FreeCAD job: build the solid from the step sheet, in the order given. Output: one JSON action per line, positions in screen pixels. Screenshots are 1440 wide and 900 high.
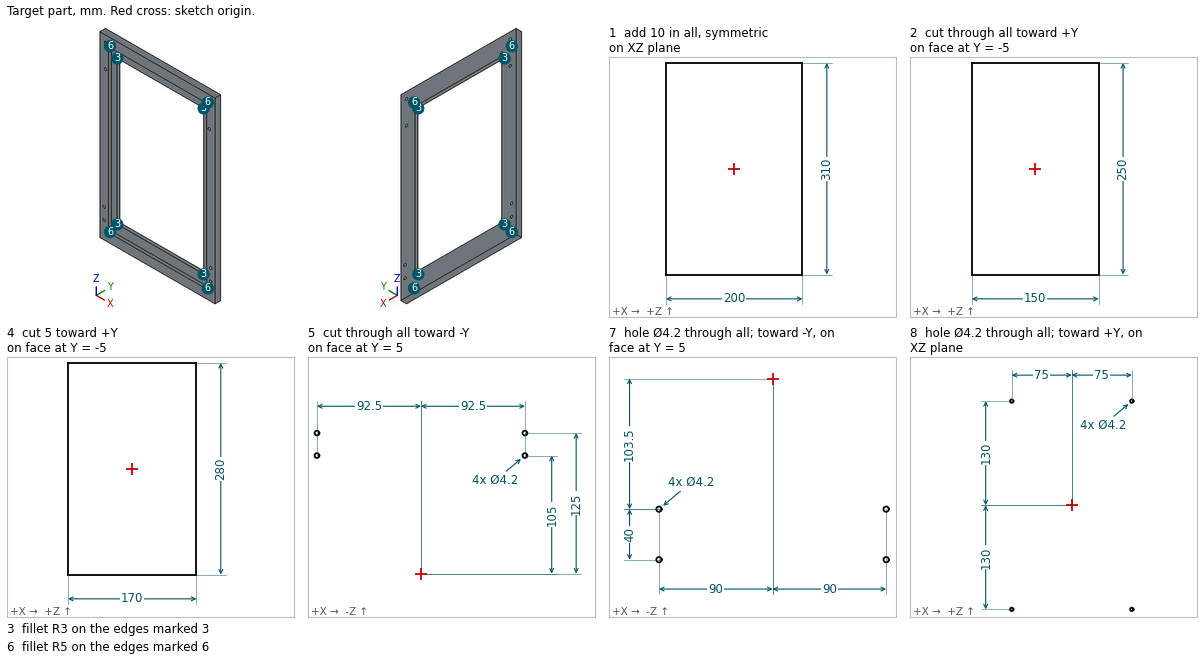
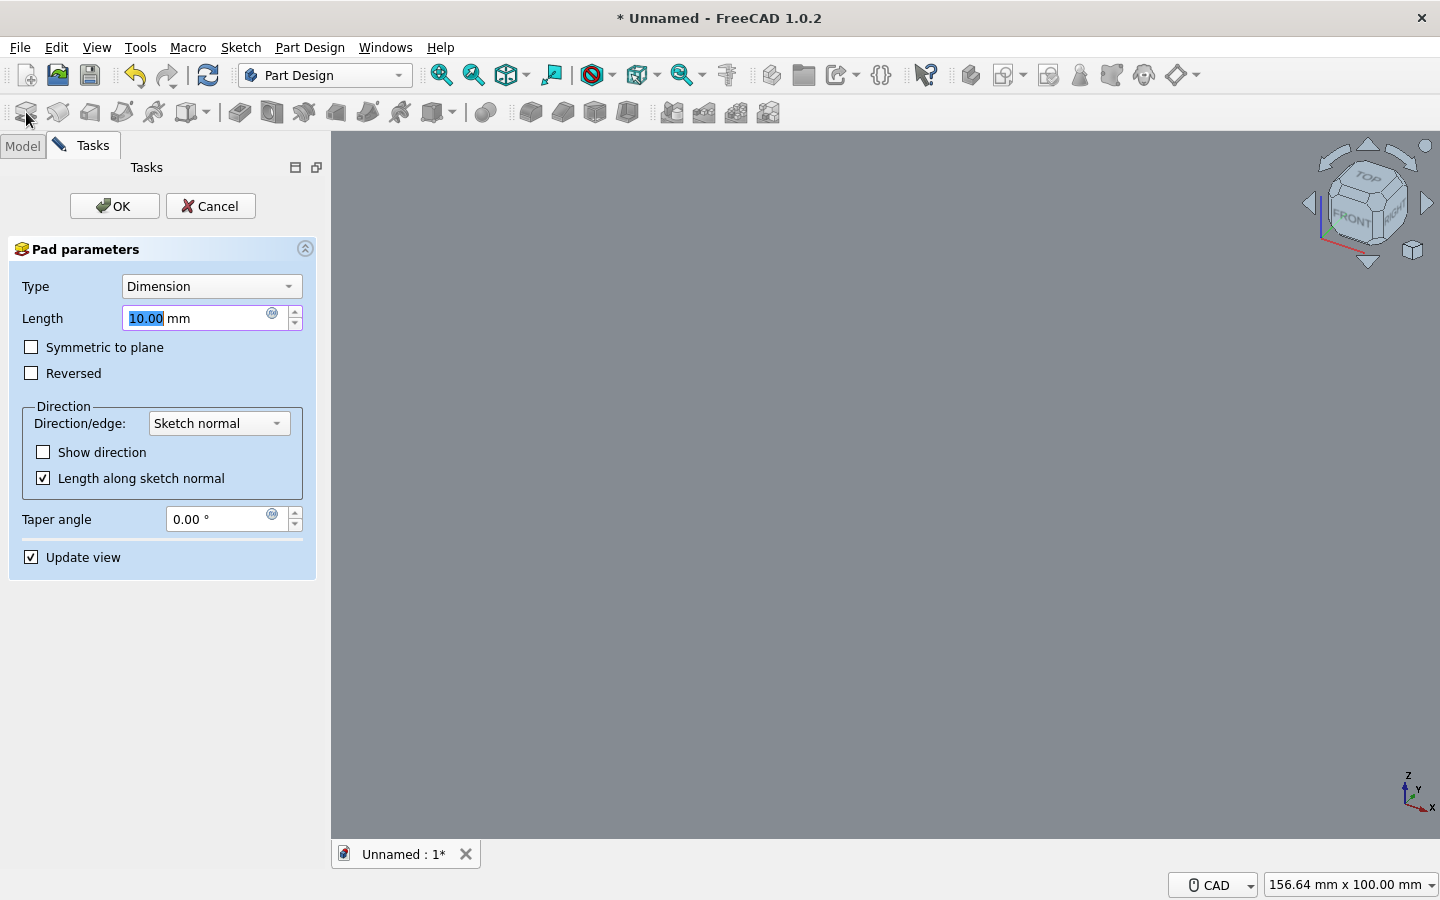
{"action": "type", "text": "10"}
{"action": "key", "text": "Tab"}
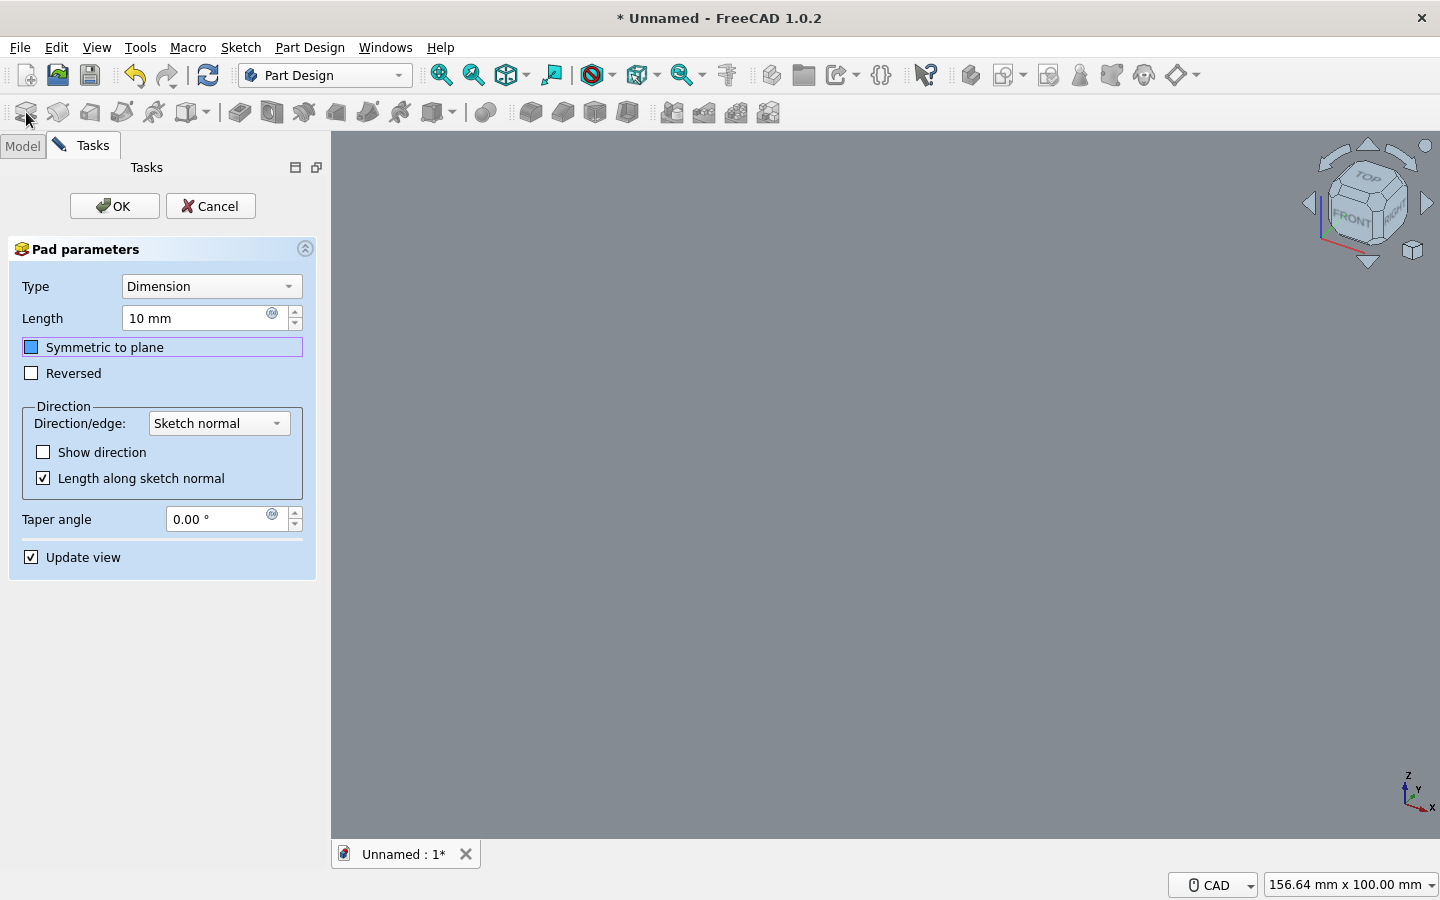
{"action": "left_click", "coordinate": [30, 347]}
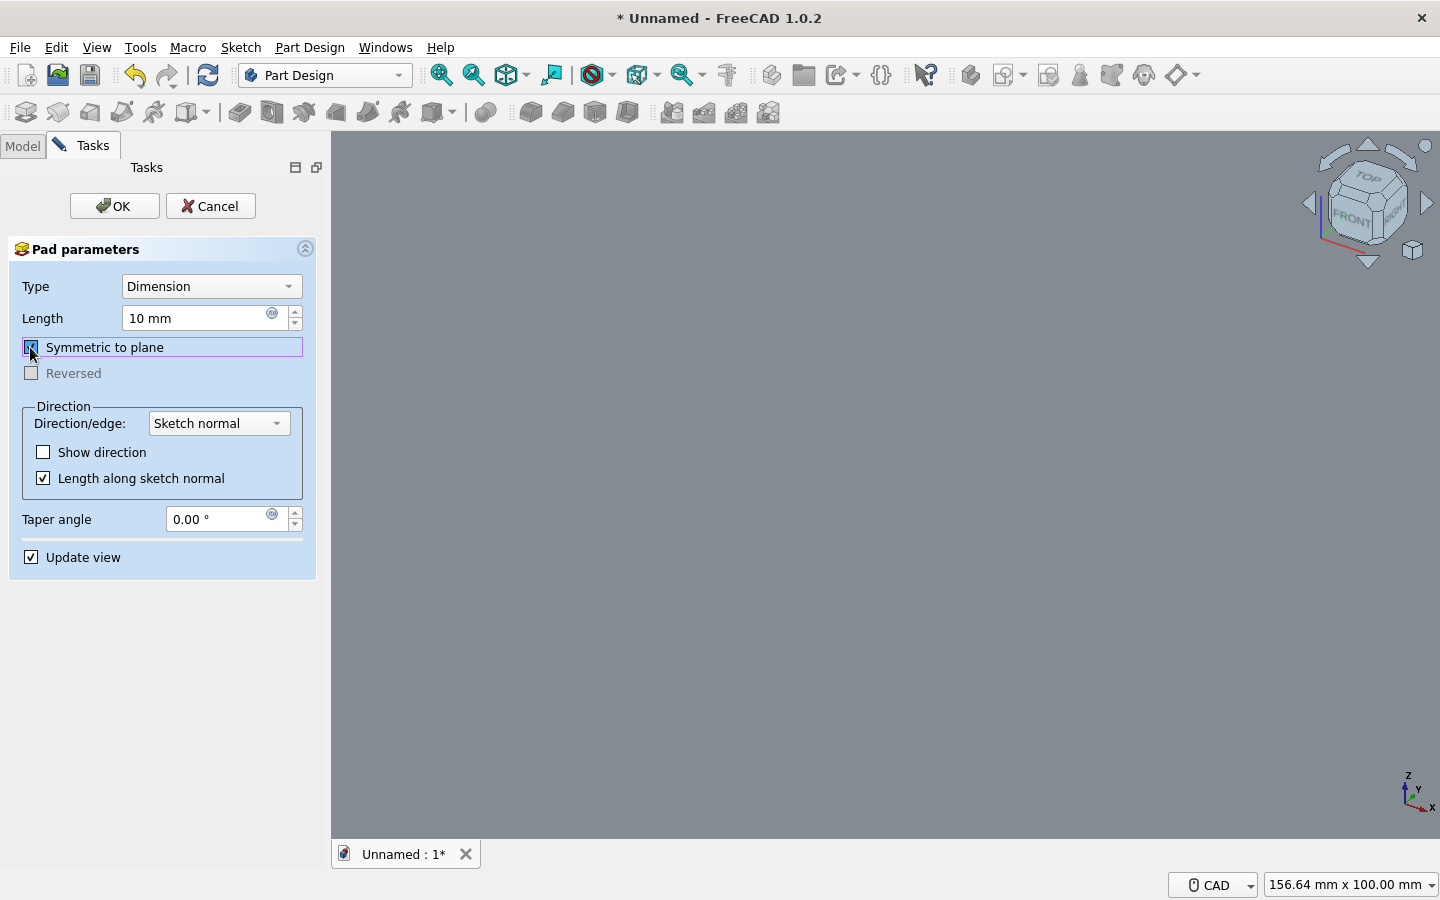
{"action": "left_click", "coordinate": [115, 206]}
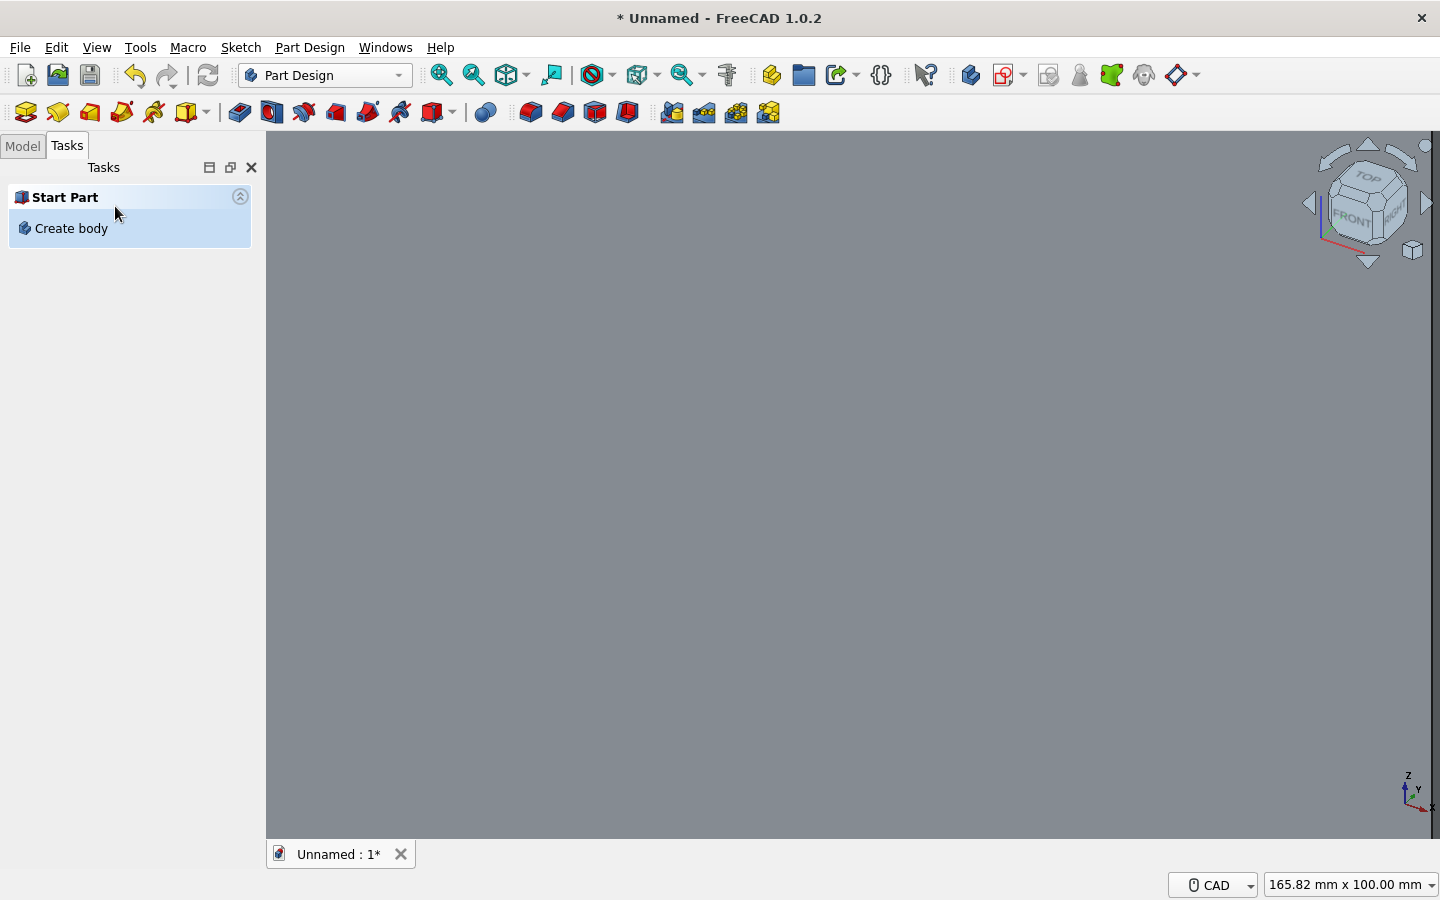
{"action": "left_click", "coordinate": [442, 76]}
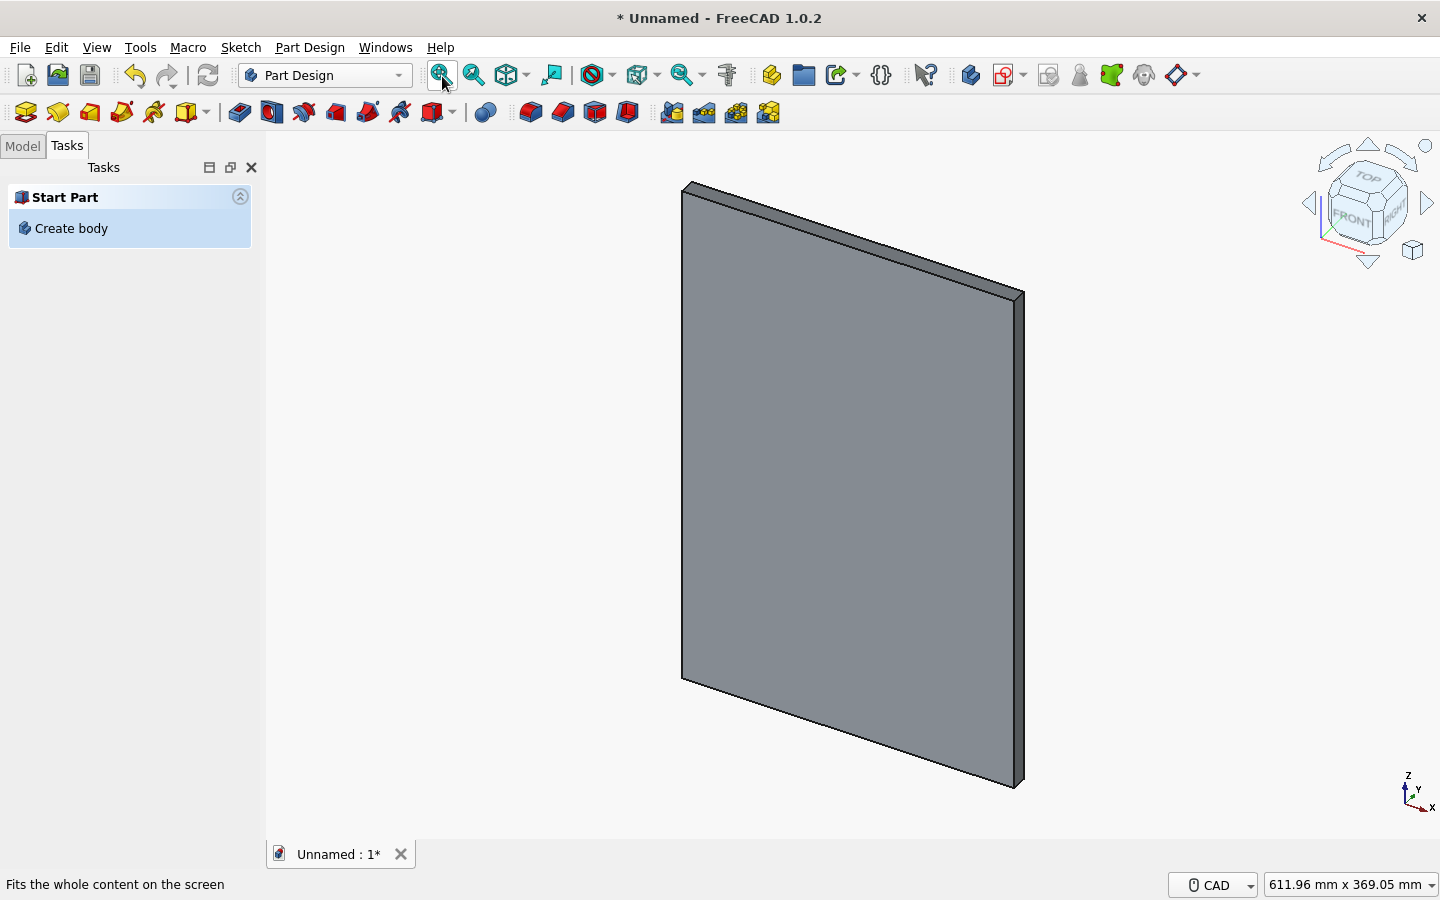
{"action": "left_click", "coordinate": [848, 419]}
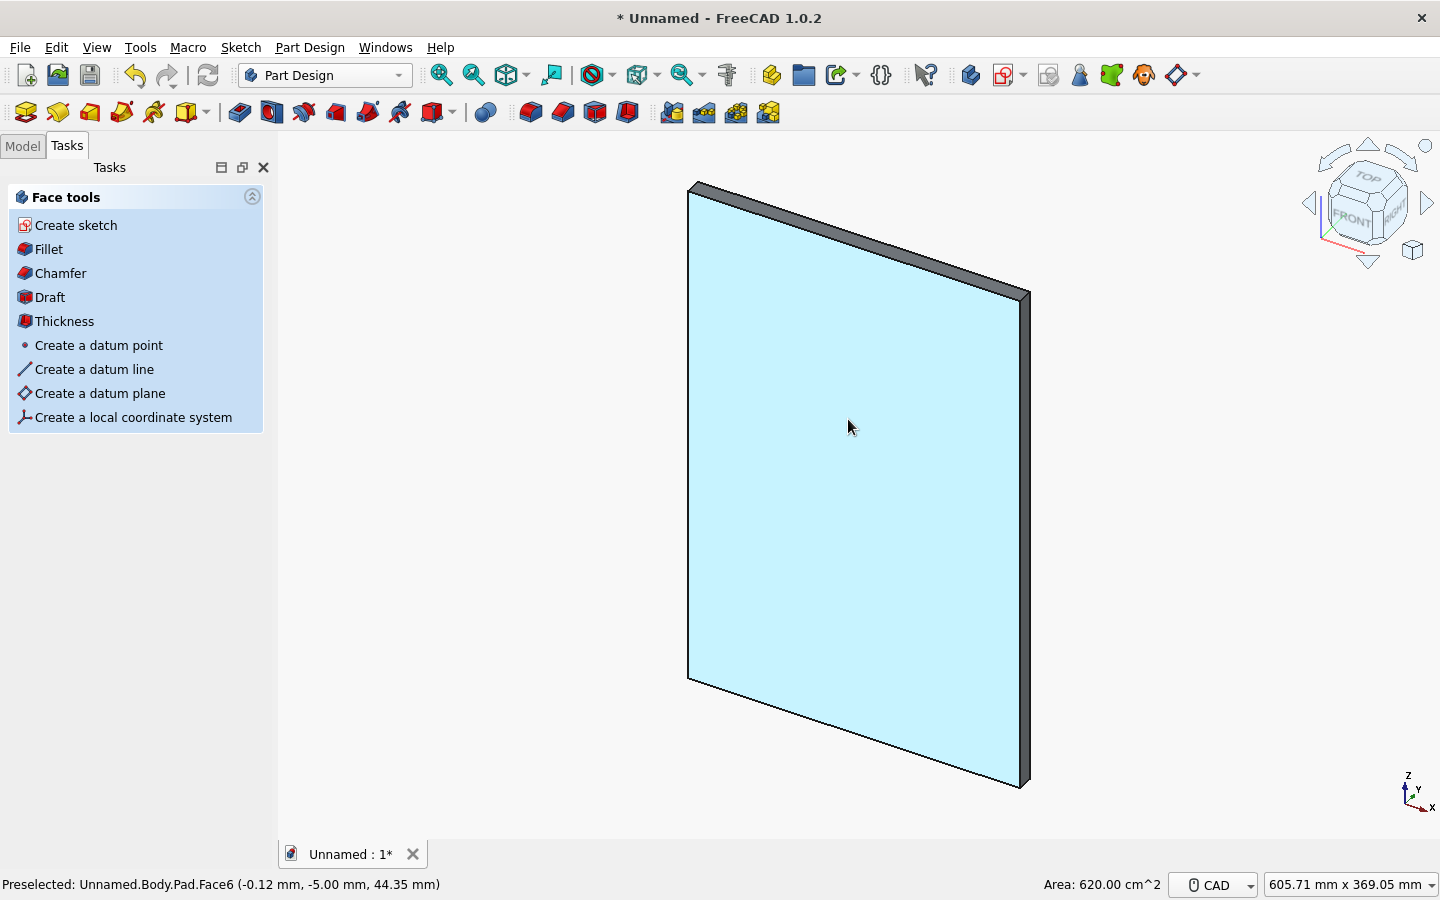
{"action": "left_click", "coordinate": [1004, 76]}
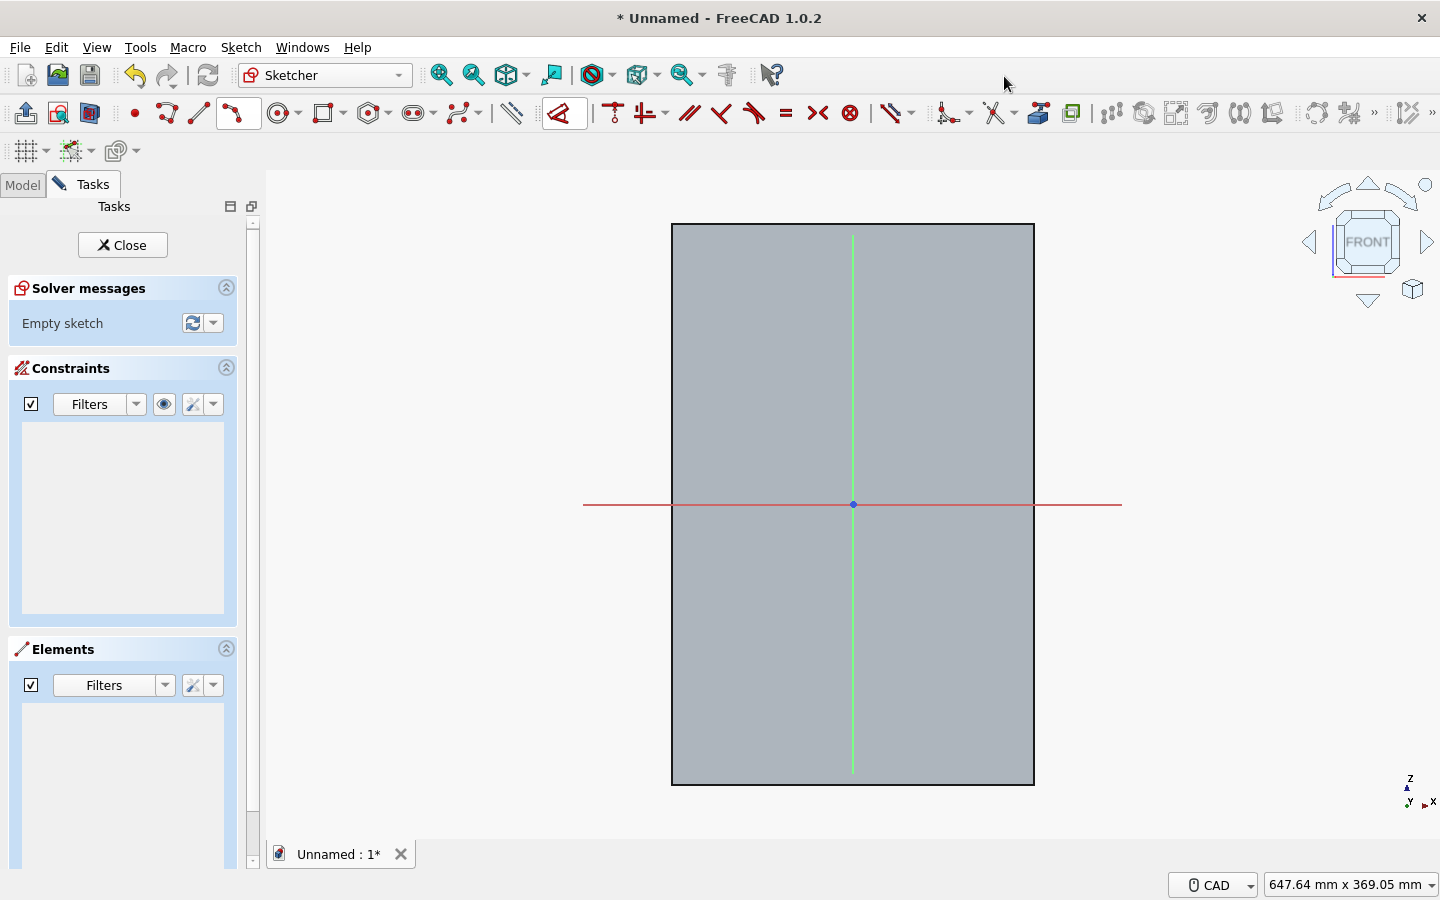
{"action": "key", "text": "g v"}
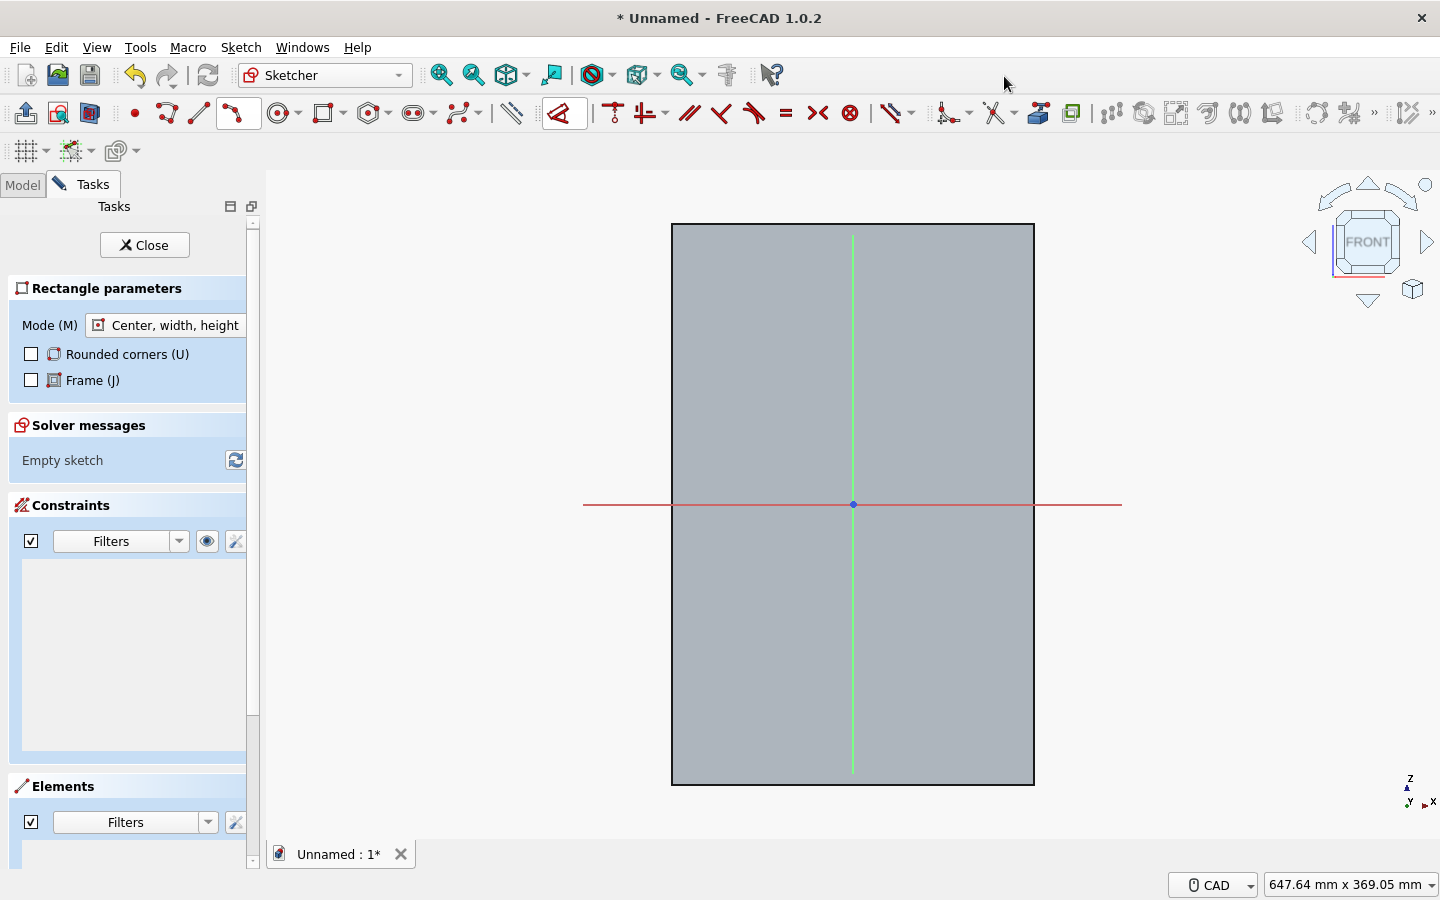
{"action": "left_click", "coordinate": [853, 504]}
{"action": "left_click", "coordinate": [989, 278]}
{"action": "key", "text": "Escape"}